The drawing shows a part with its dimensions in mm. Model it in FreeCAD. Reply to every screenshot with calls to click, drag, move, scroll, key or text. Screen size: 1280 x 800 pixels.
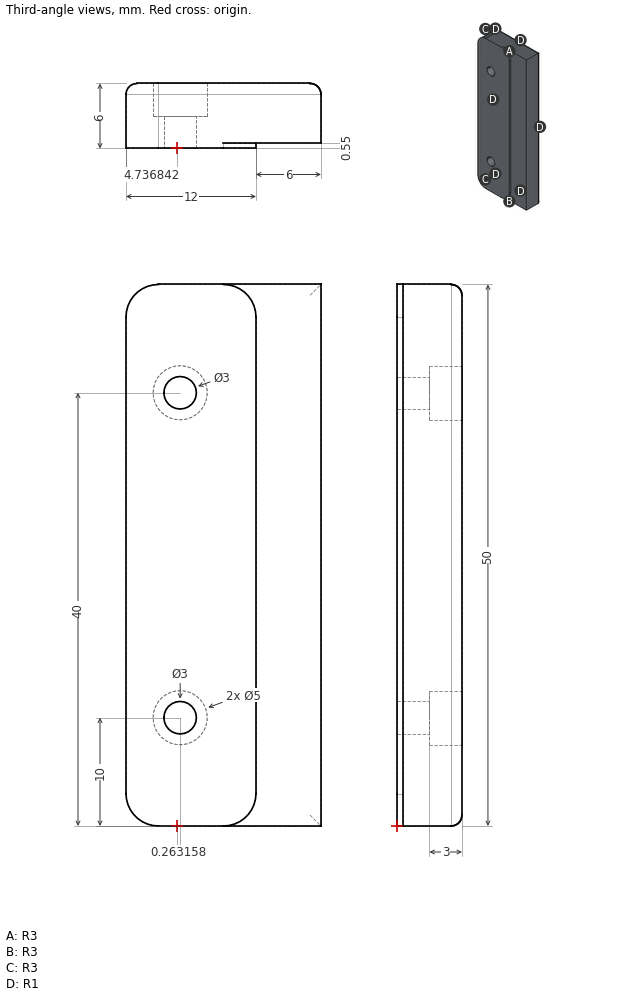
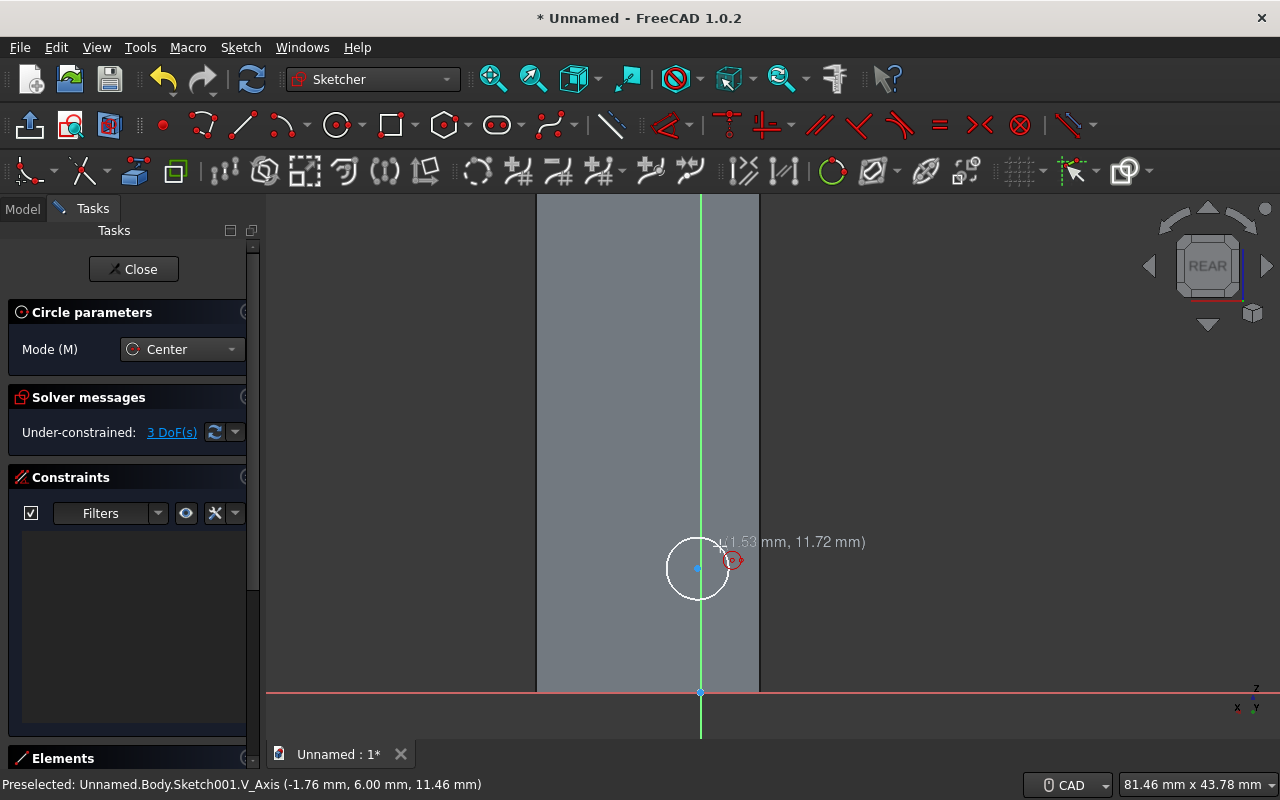
scroll(718, 544, down, 2)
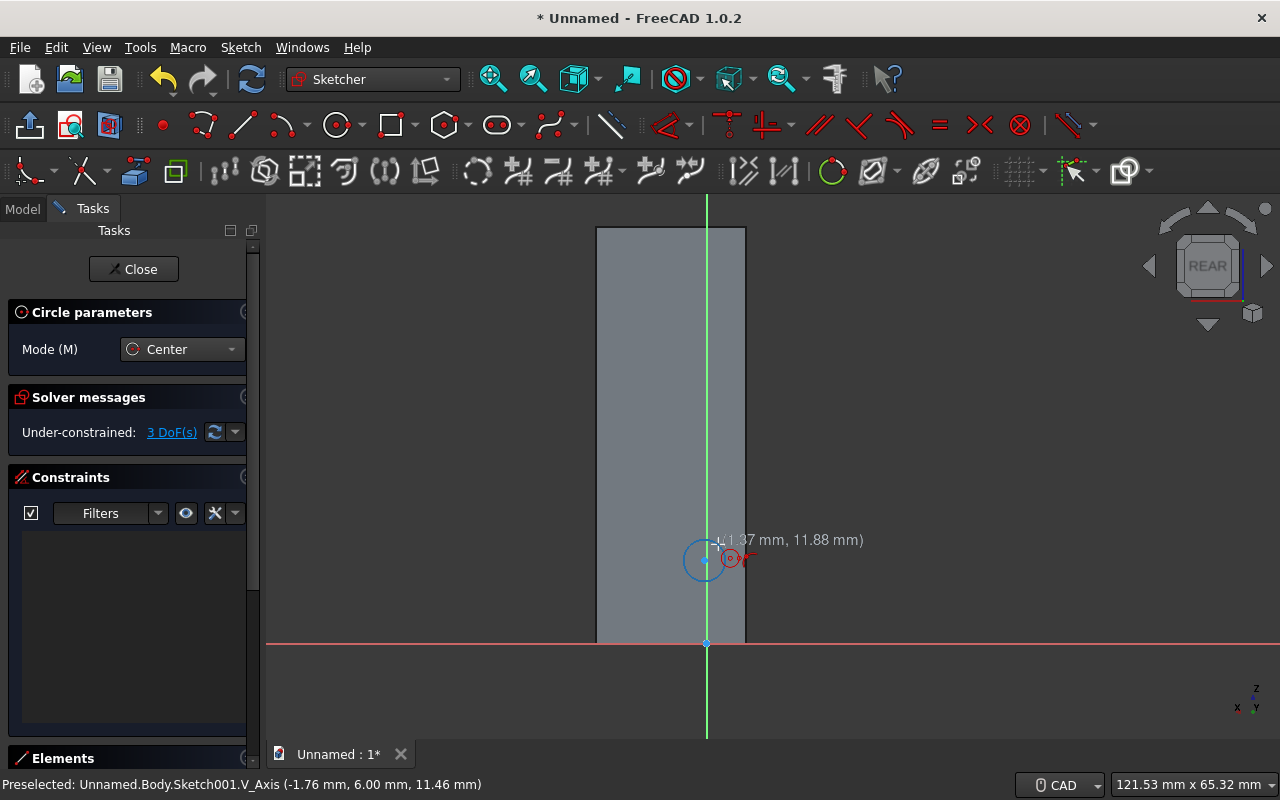
scroll(704, 310, up, 10)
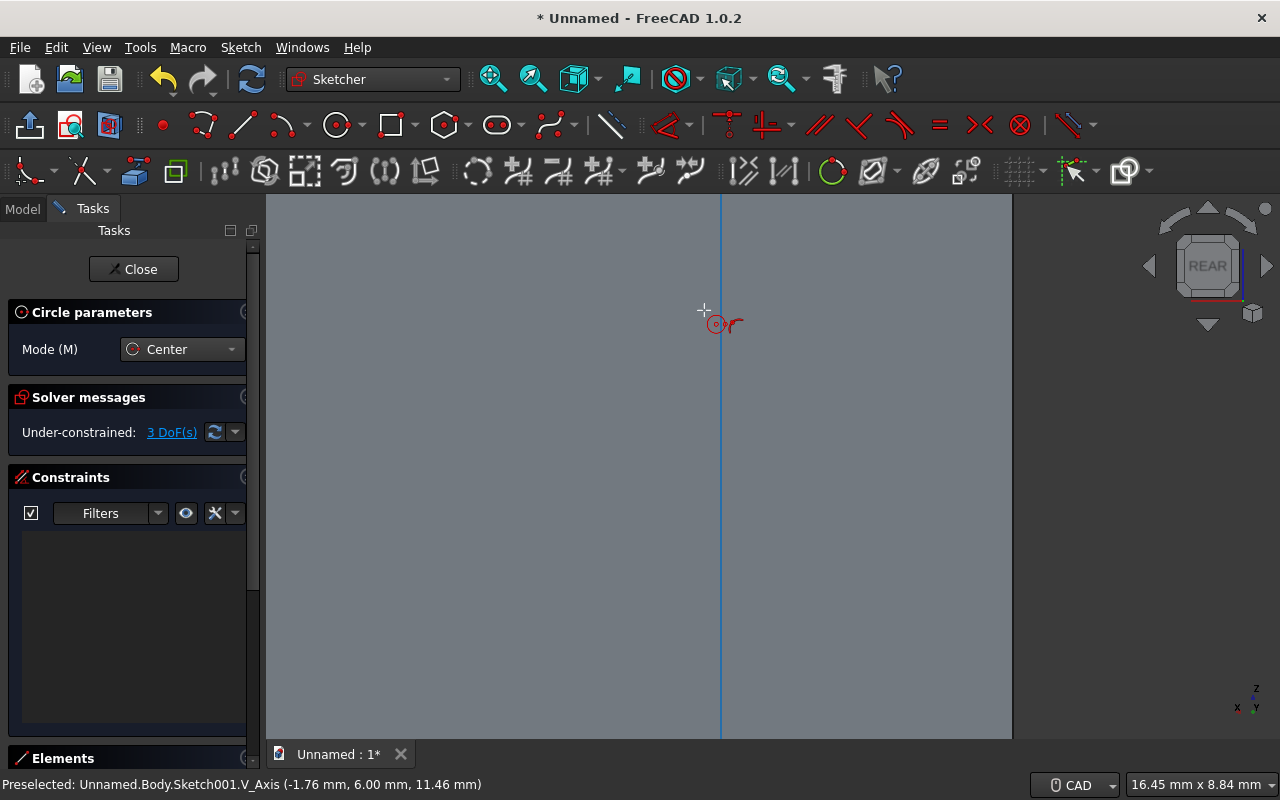
click(705, 310)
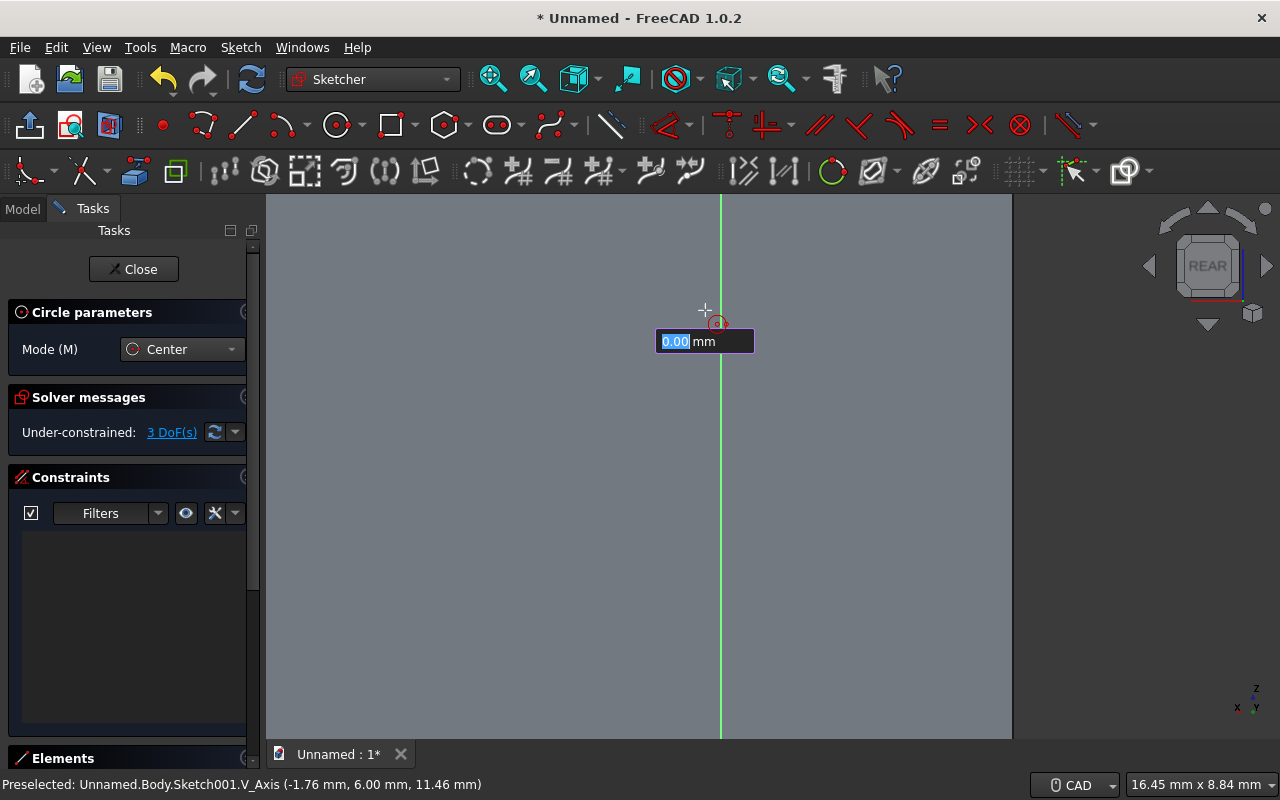
scroll(704, 310, down, 10)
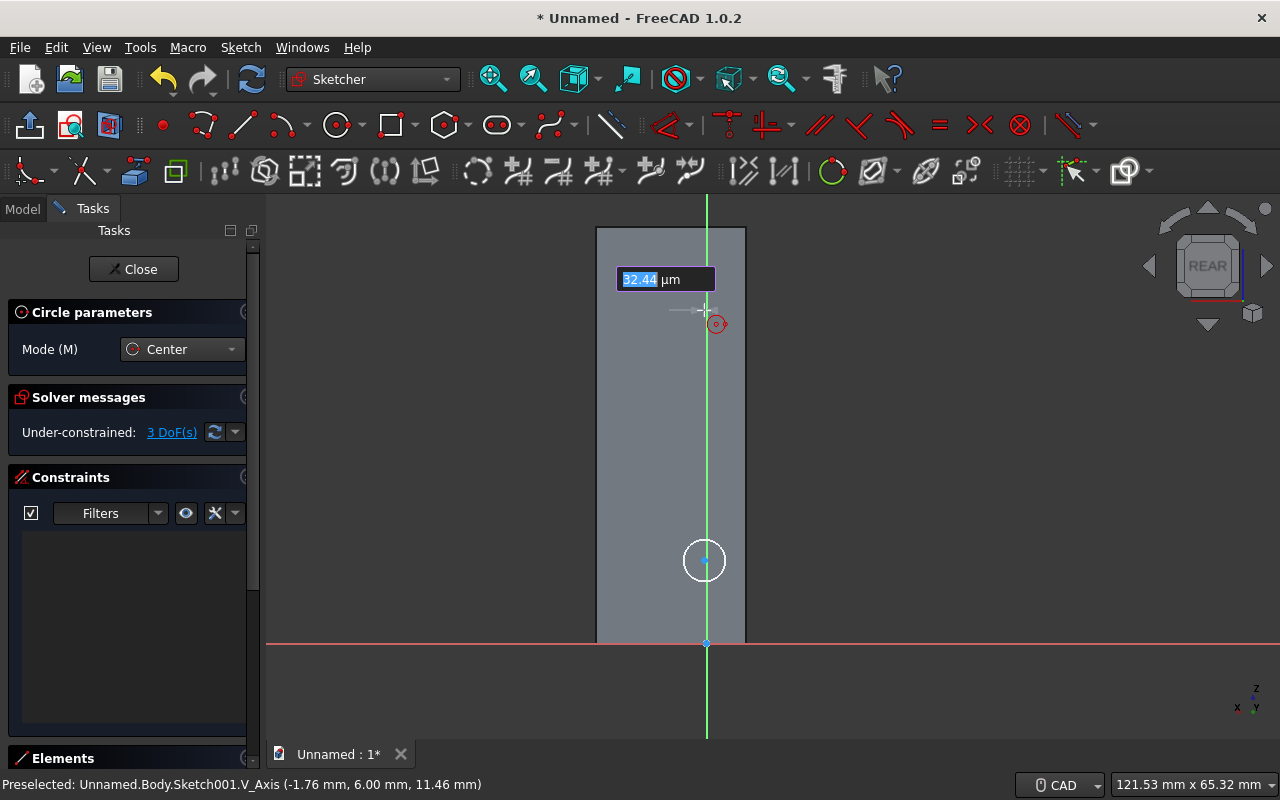
scroll(719, 295, up, 2)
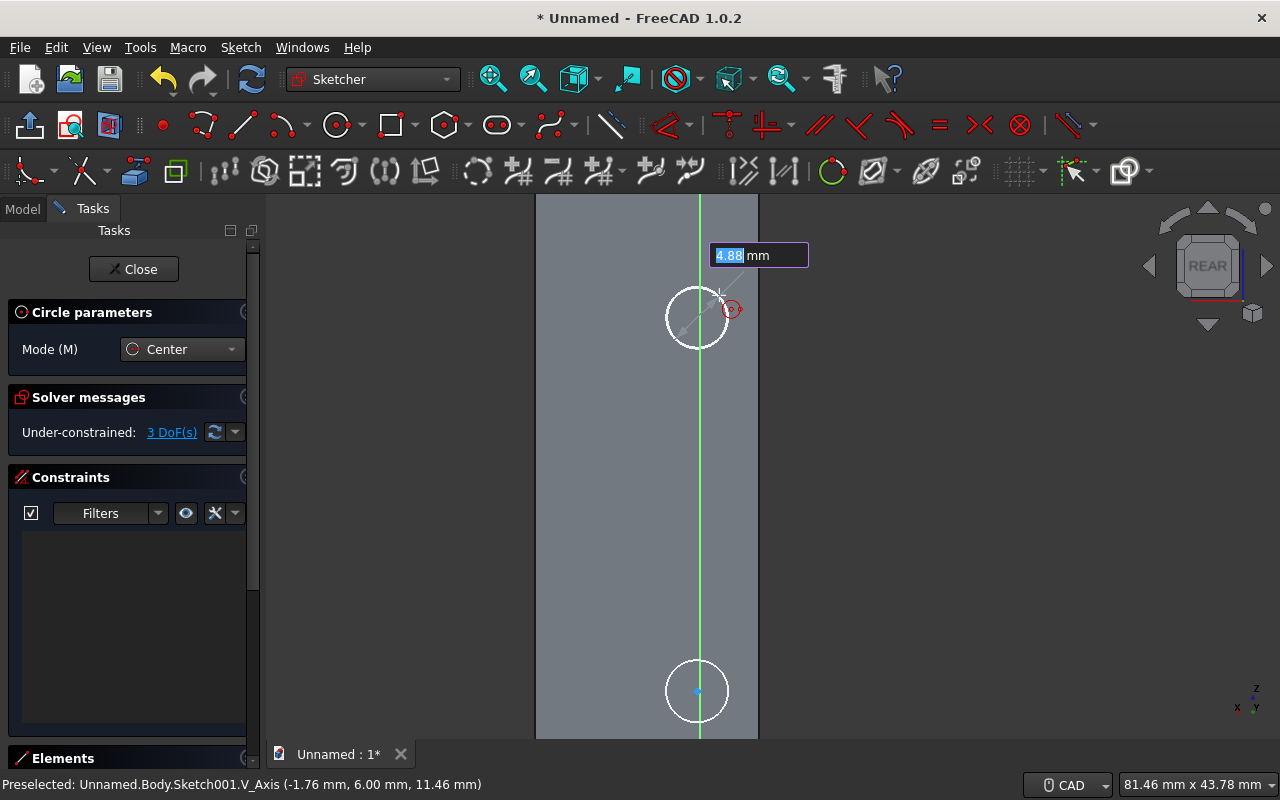
click(719, 296)
key(Escape)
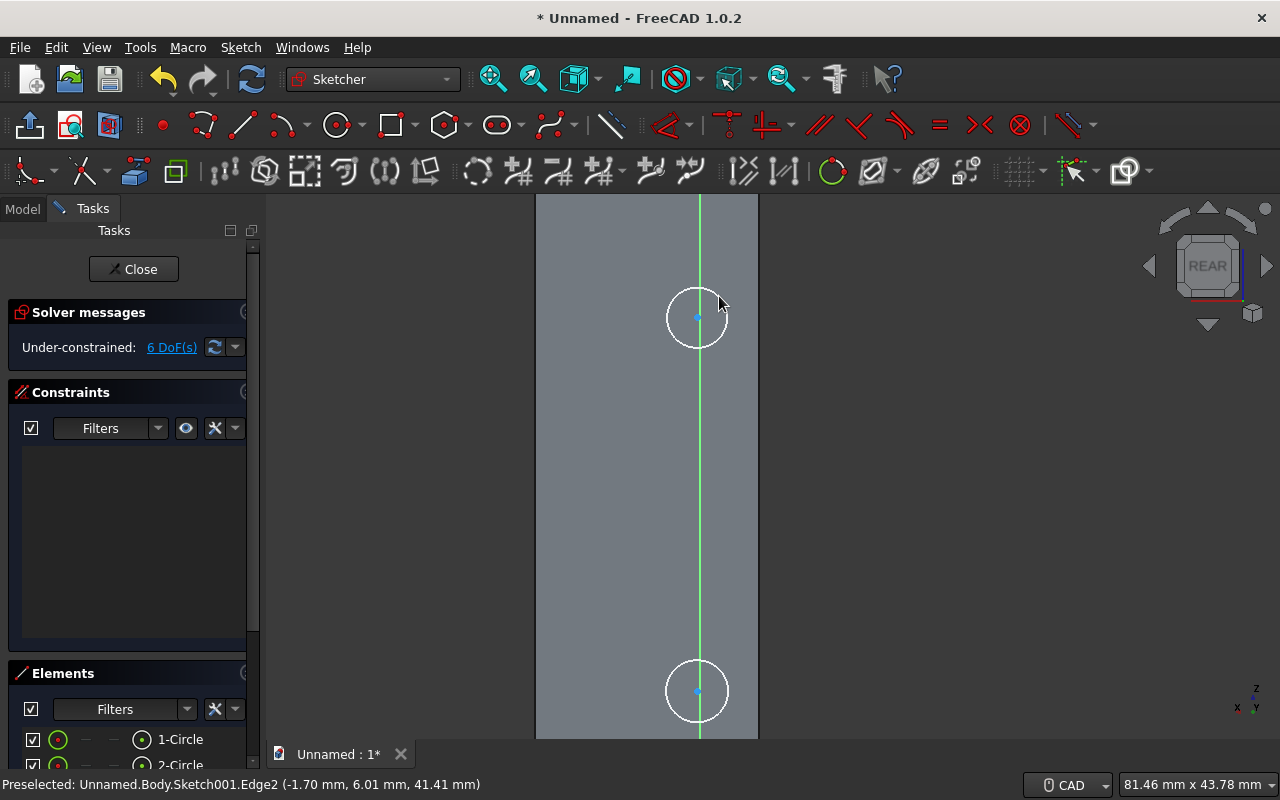
click(719, 669)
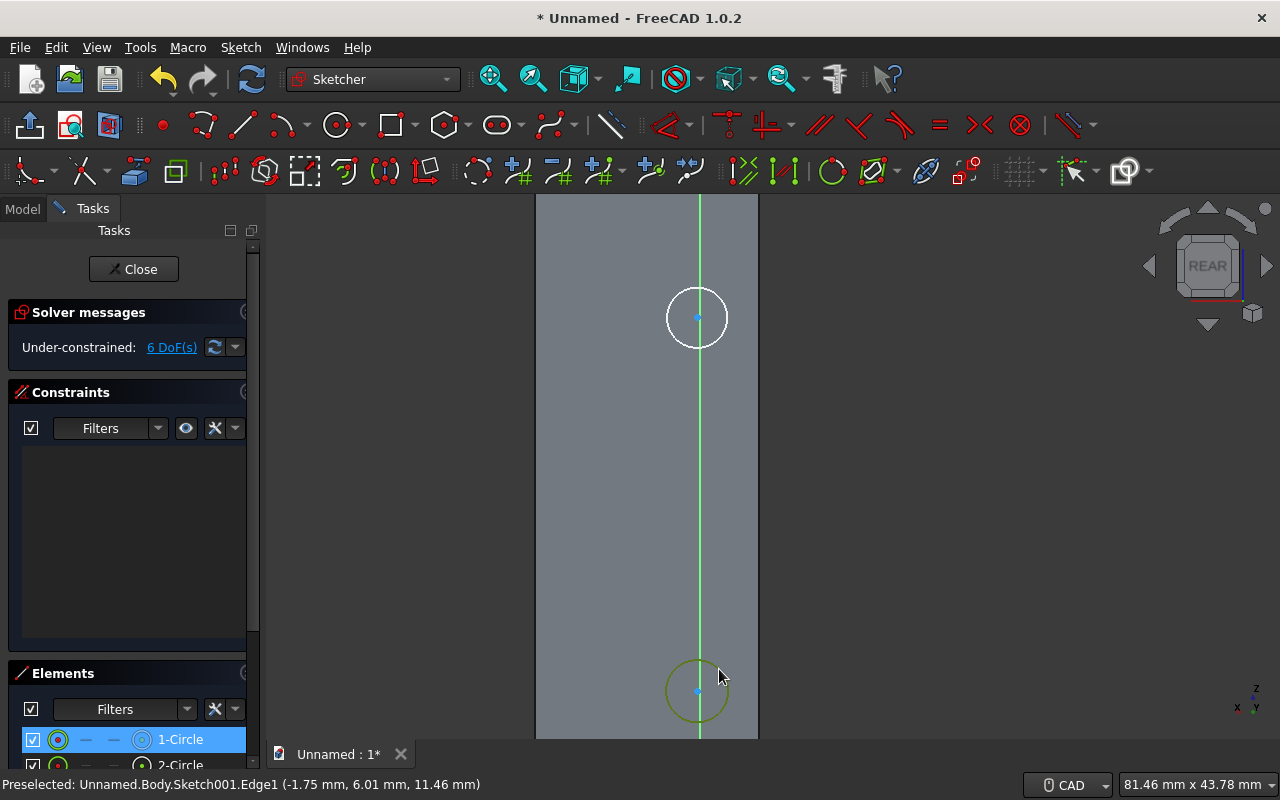
click(718, 296)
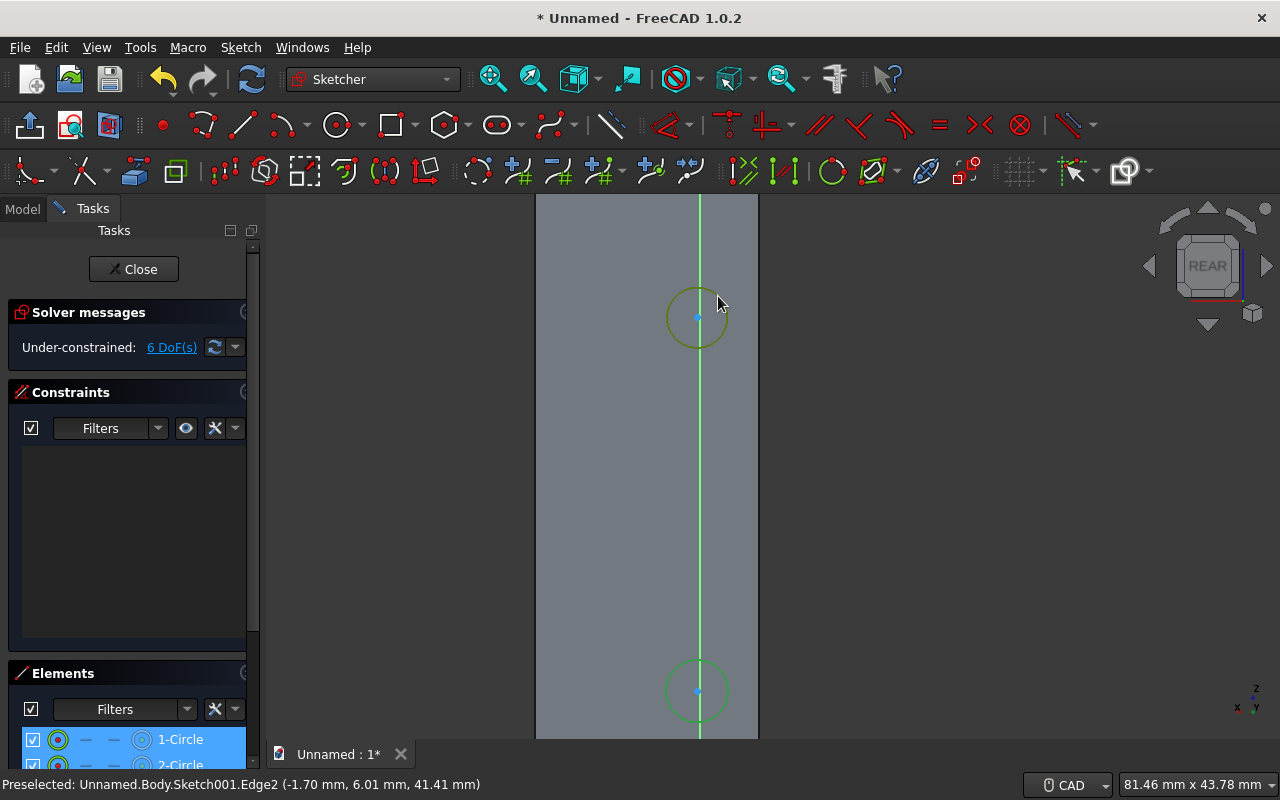
click(940, 126)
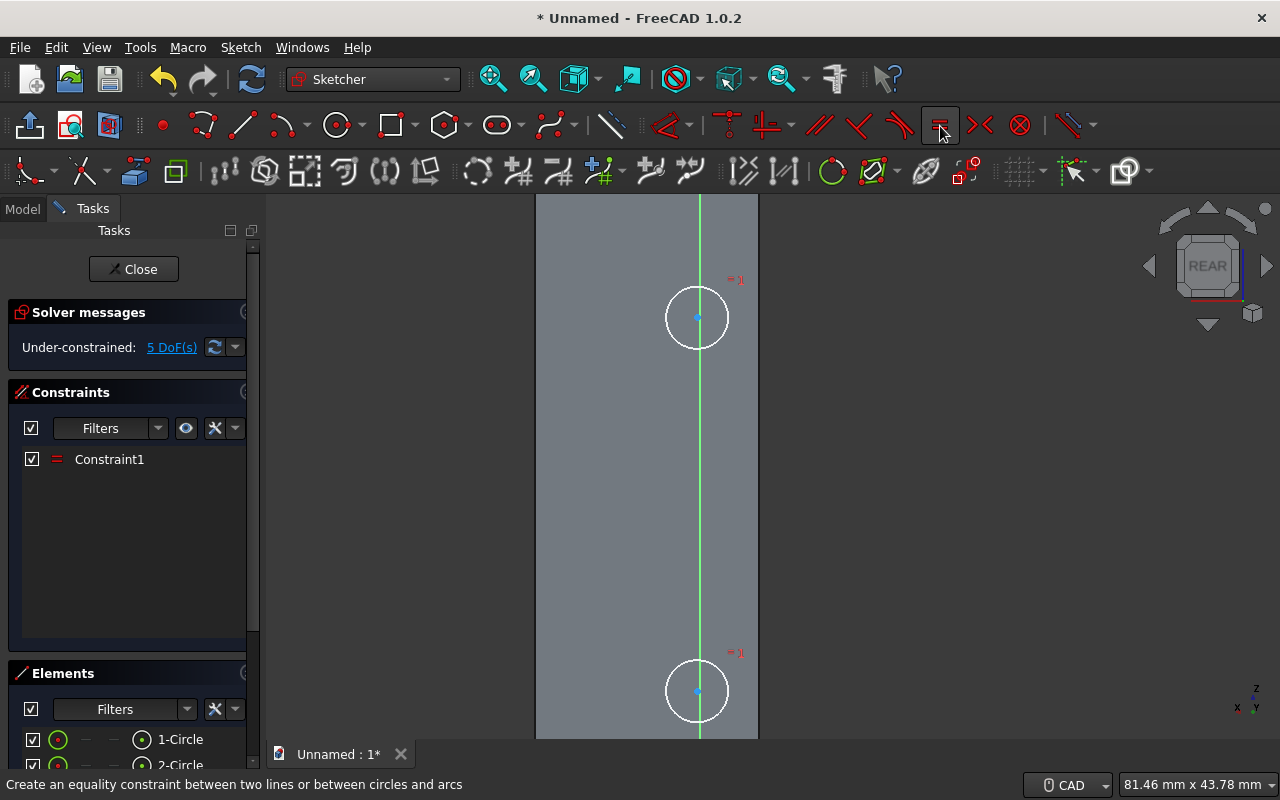
key(d)